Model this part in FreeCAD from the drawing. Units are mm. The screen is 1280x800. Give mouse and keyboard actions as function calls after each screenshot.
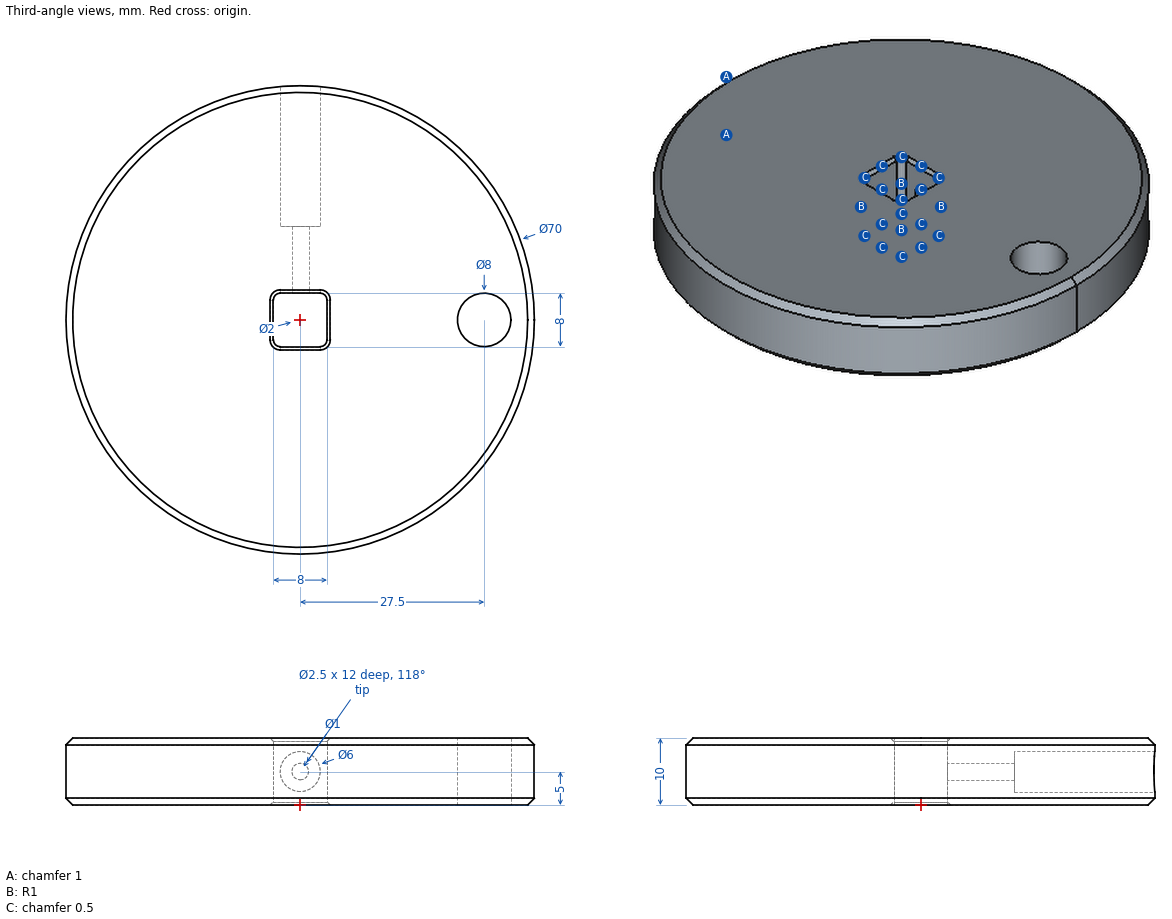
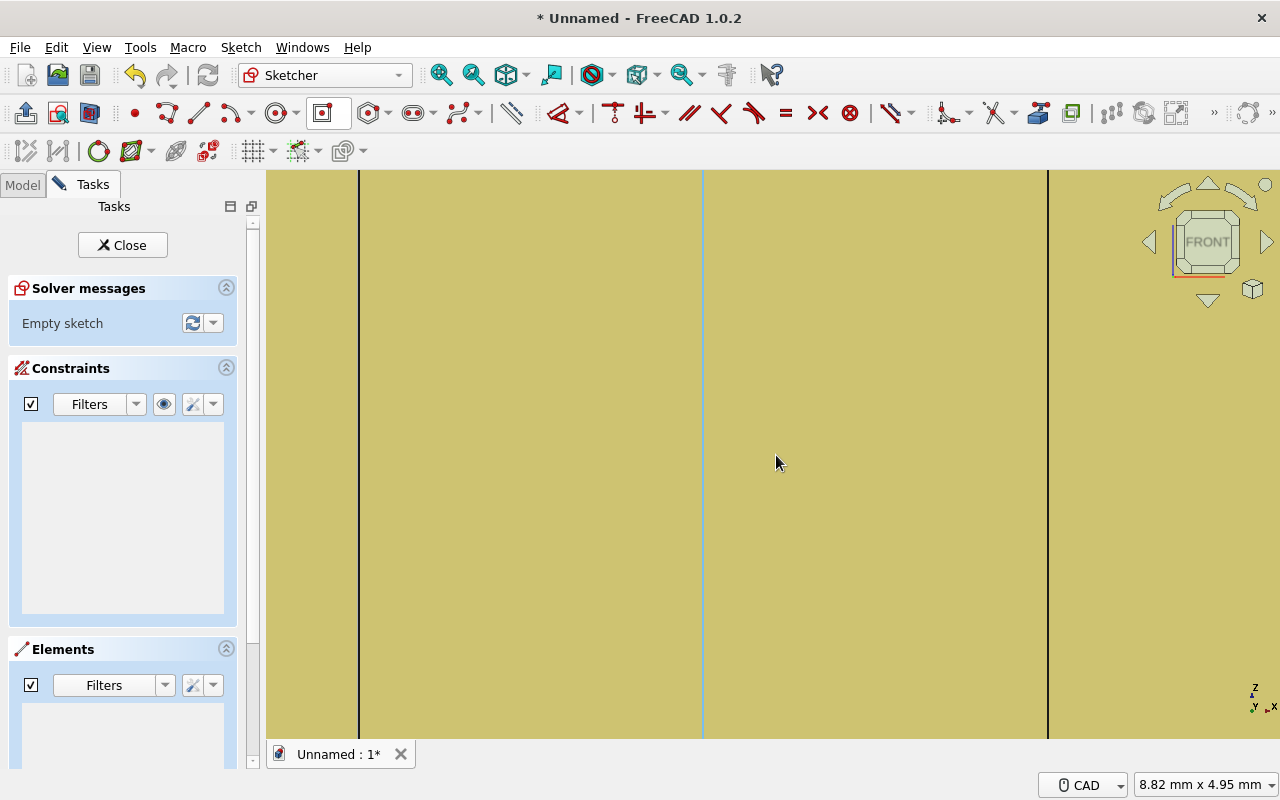
scroll(703, 427, up, 6)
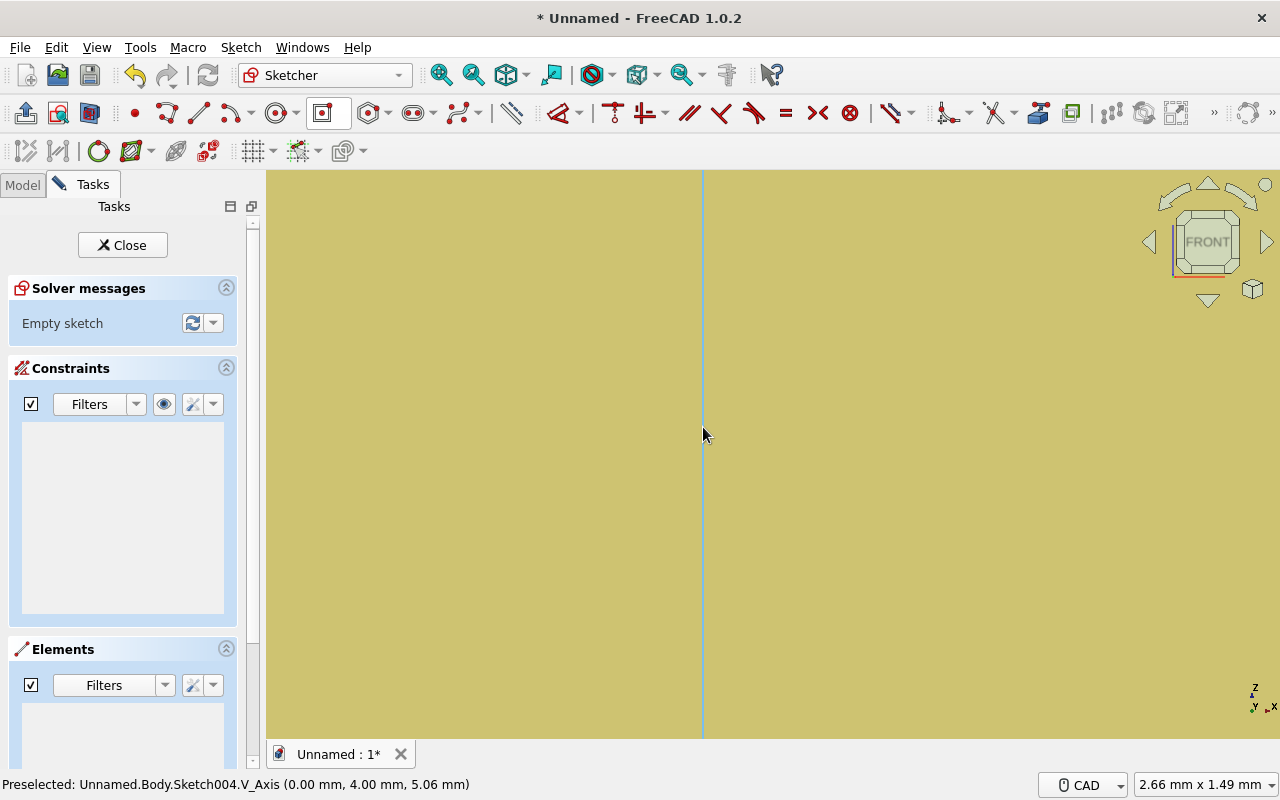
click(276, 114)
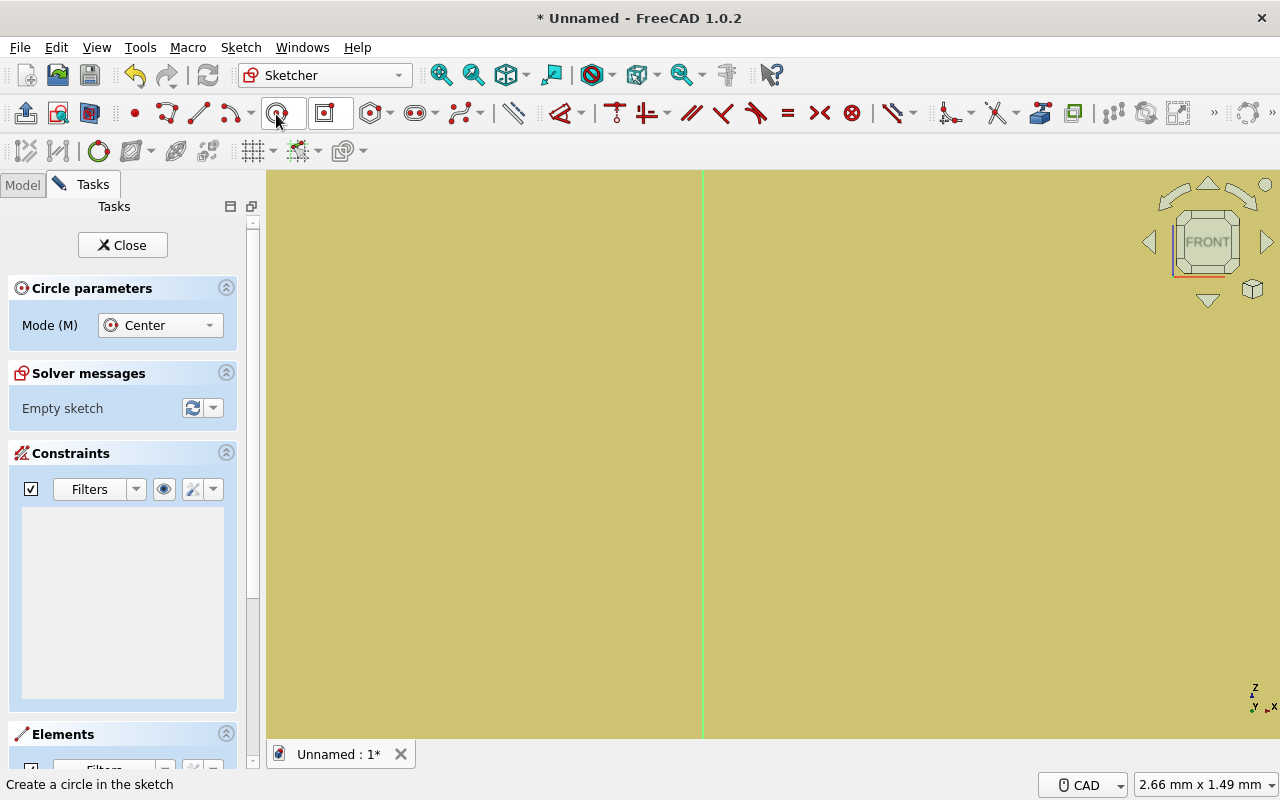
click(703, 454)
click(838, 319)
key(Escape)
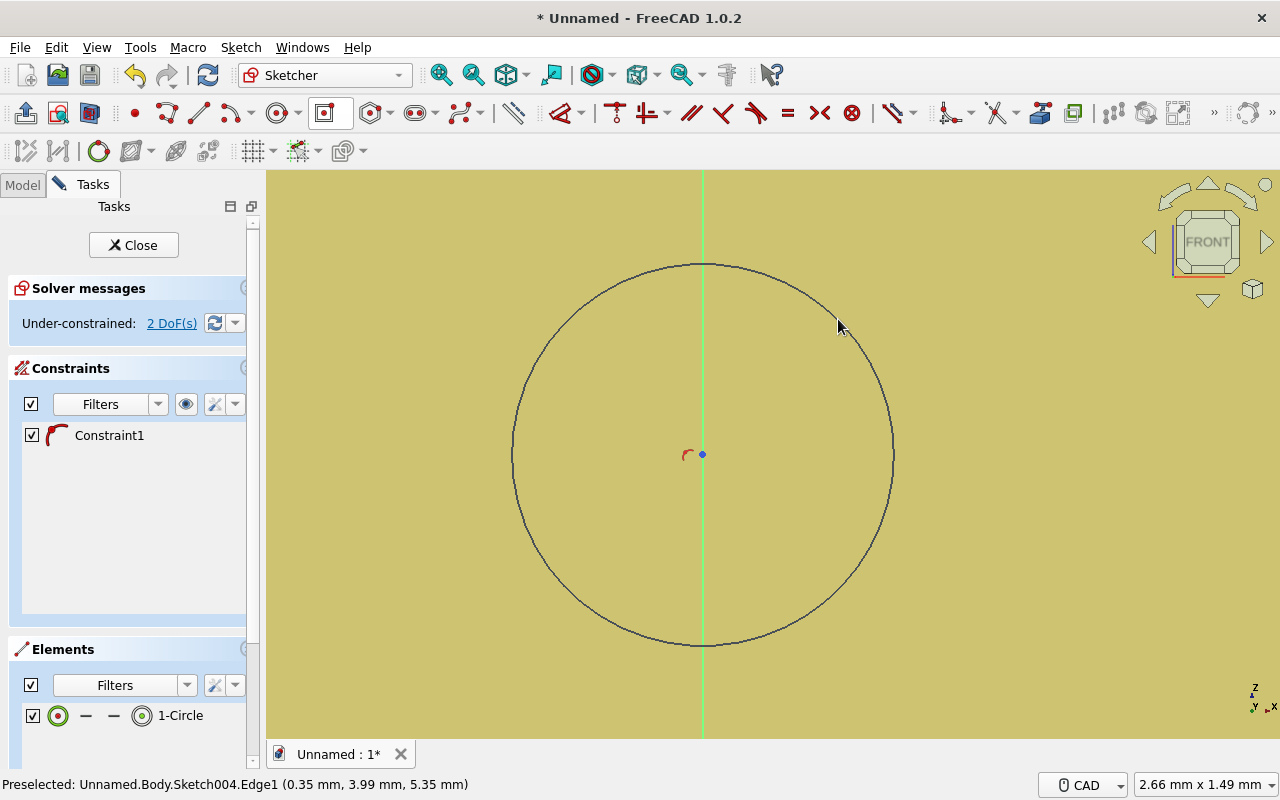
key(d)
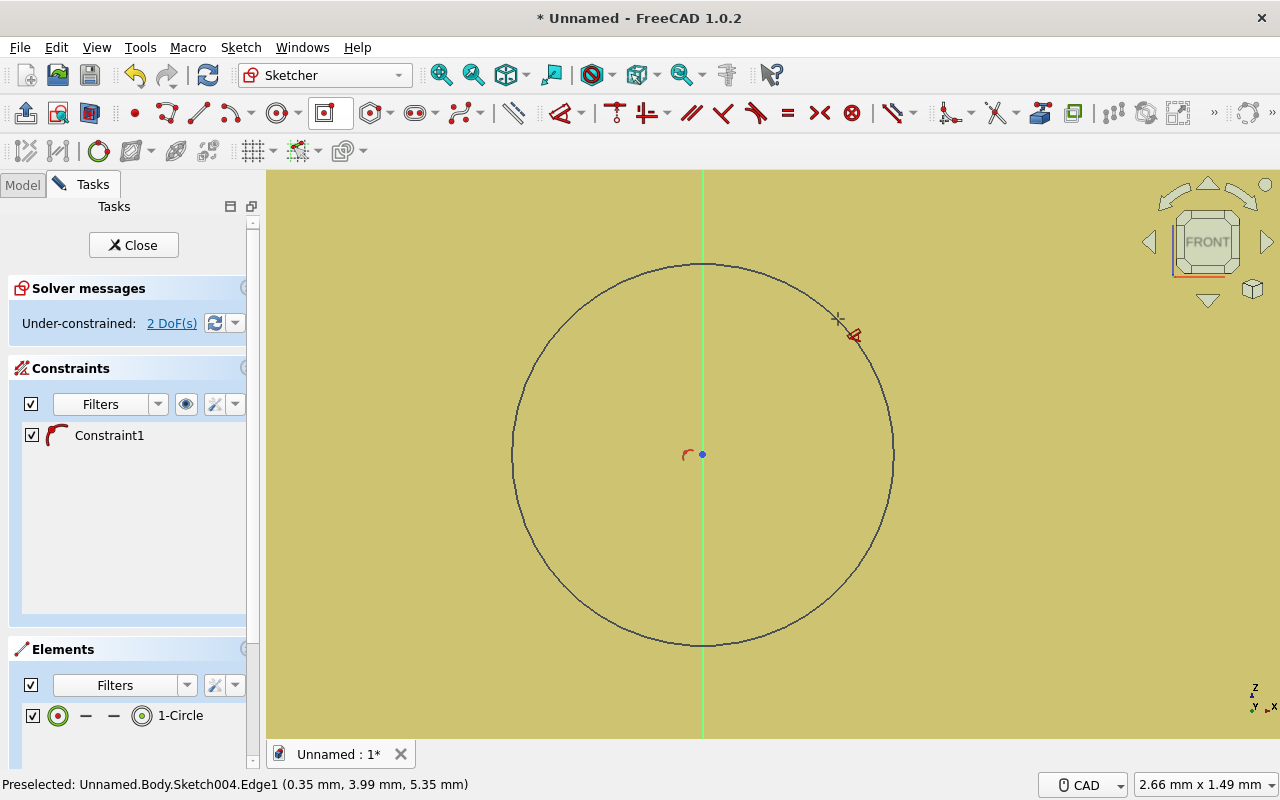
click(838, 320)
click(861, 297)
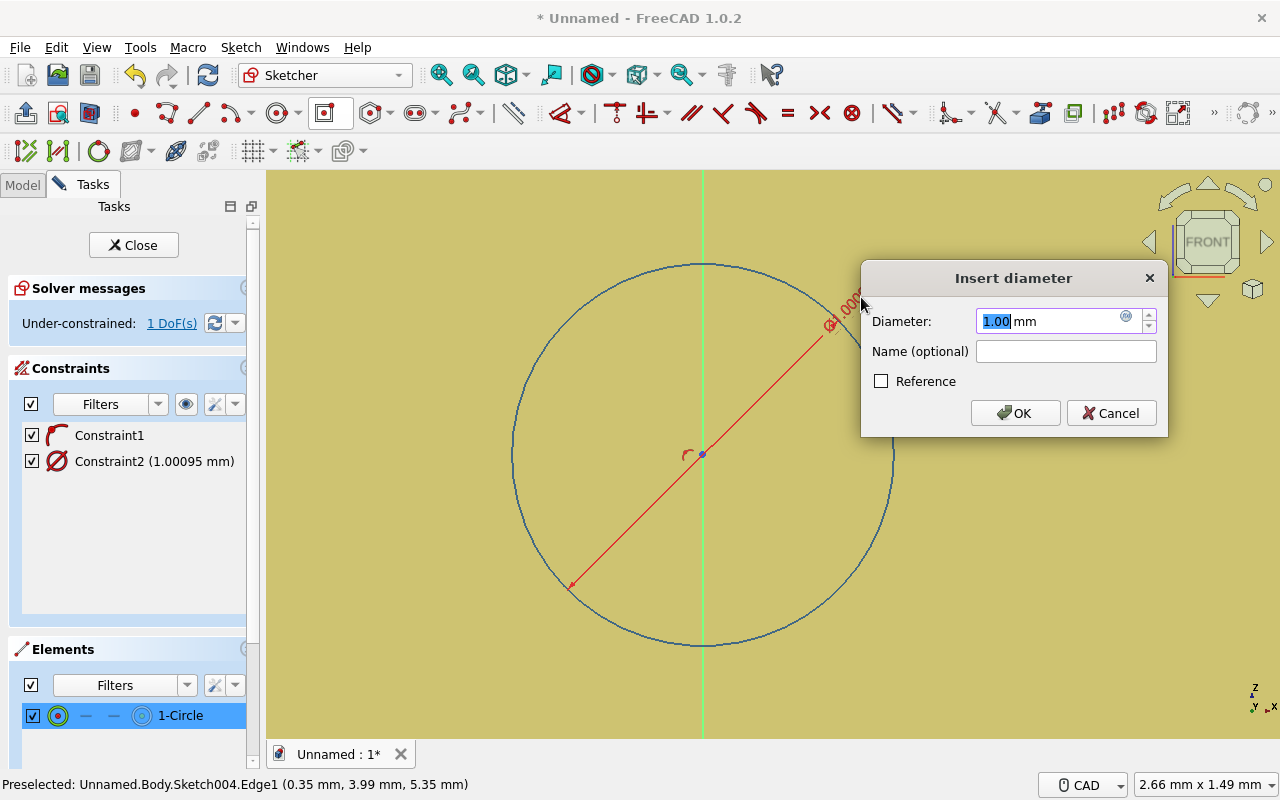
text(1)
key(Return)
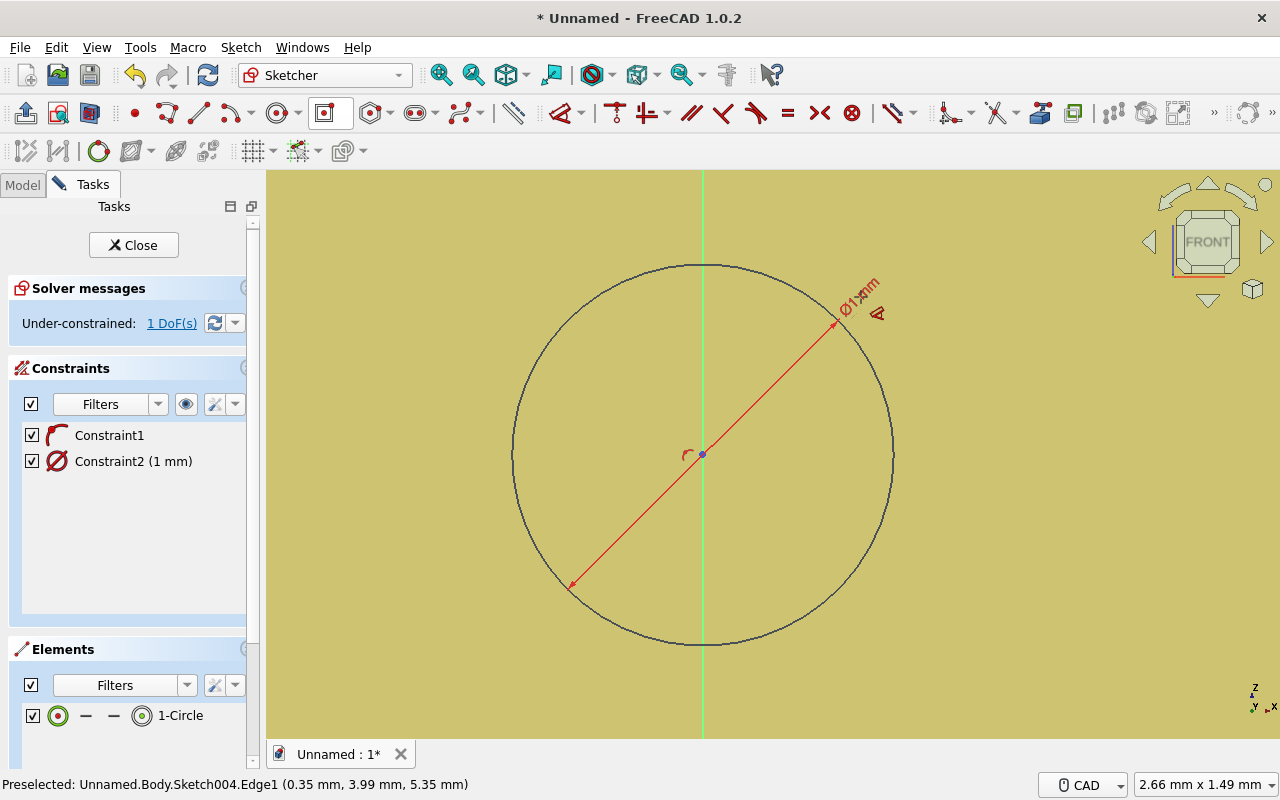
click(703, 455)
click(737, 583)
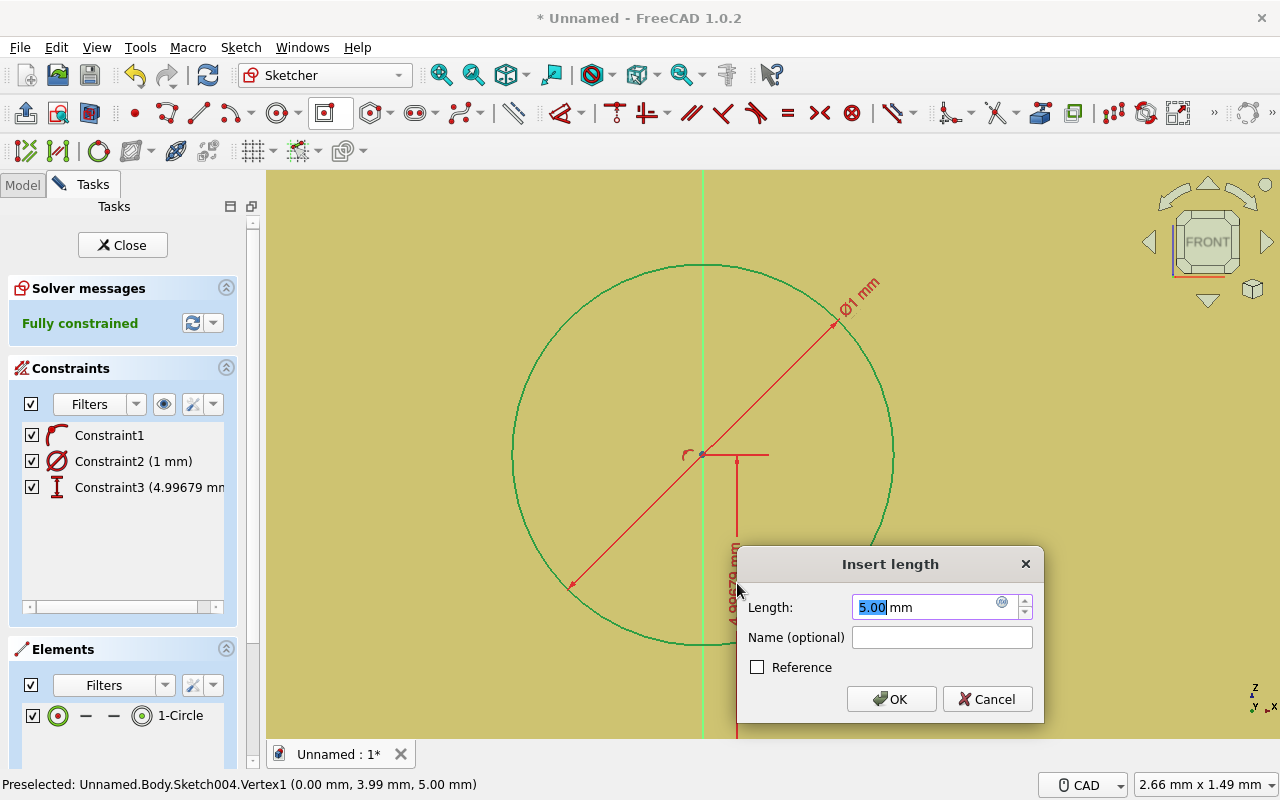
text(5)
key(Return)
key(Escape)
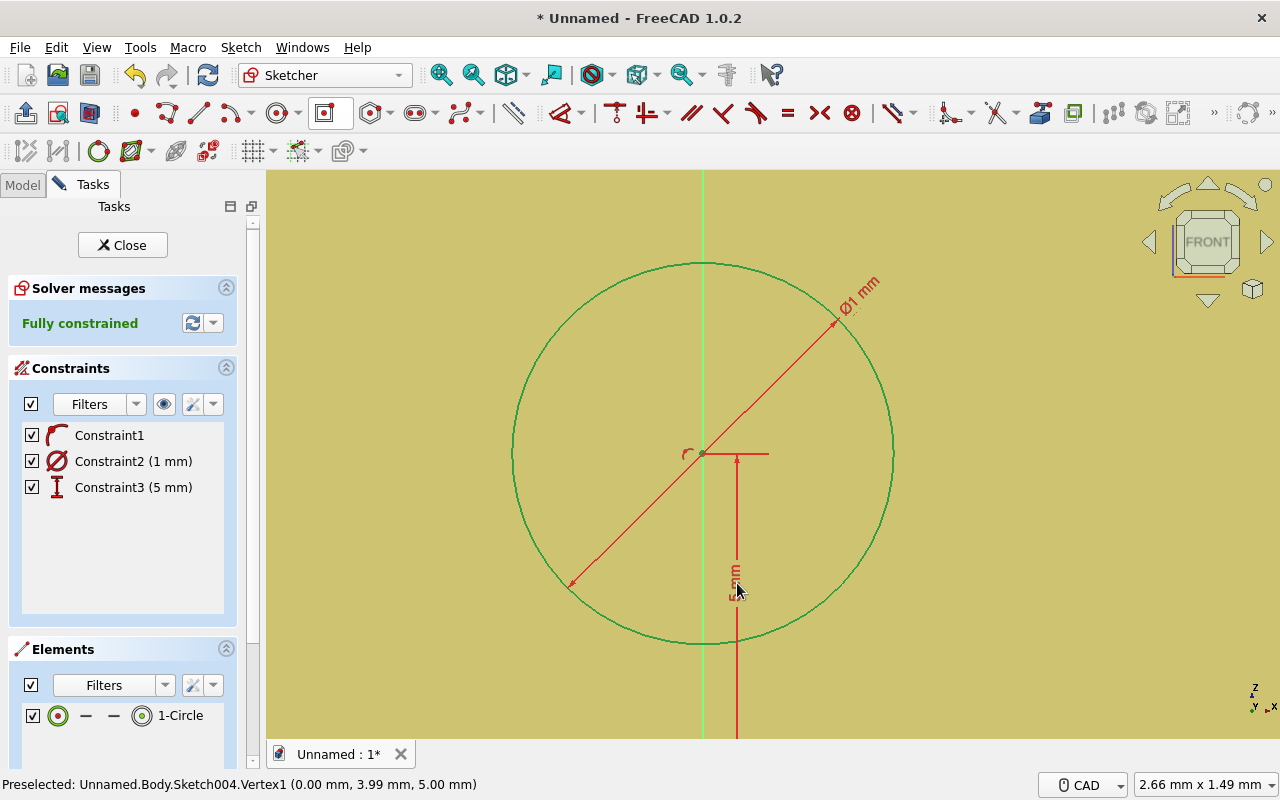
click(123, 245)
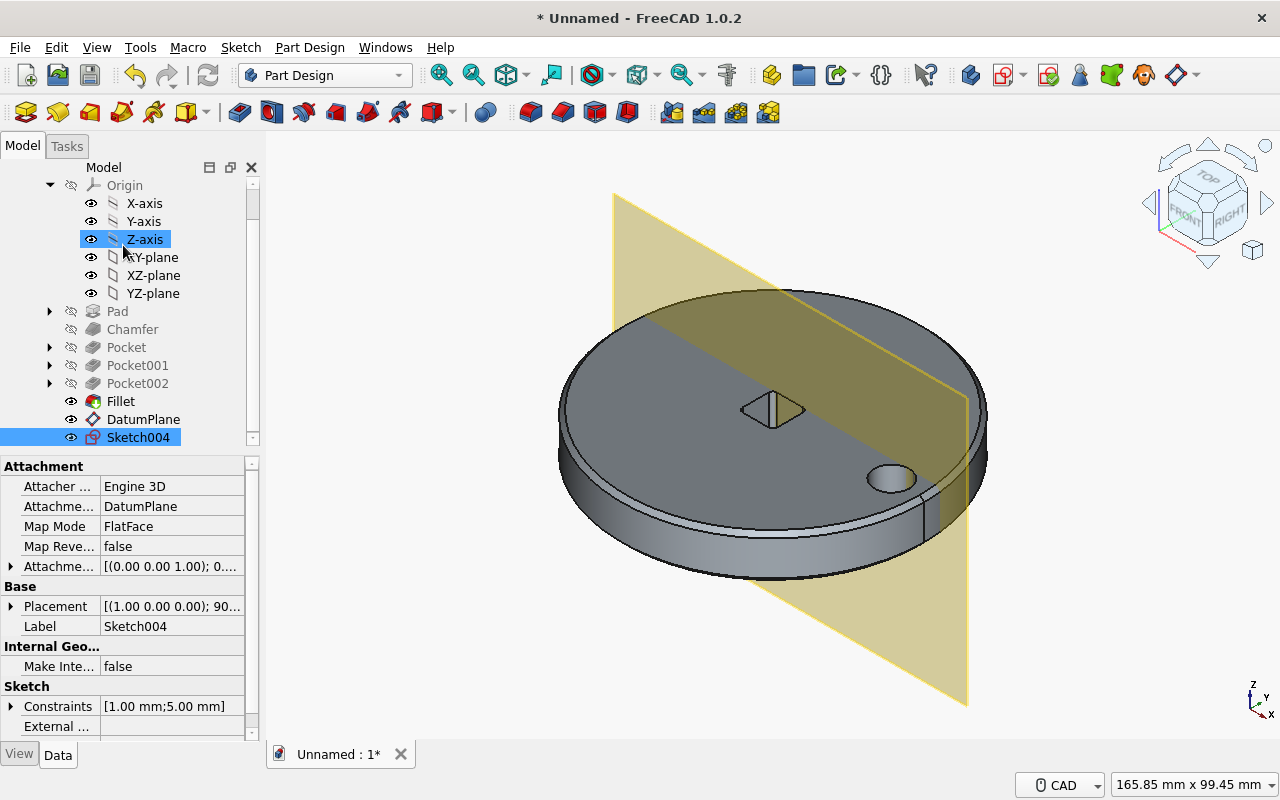
click(240, 112)